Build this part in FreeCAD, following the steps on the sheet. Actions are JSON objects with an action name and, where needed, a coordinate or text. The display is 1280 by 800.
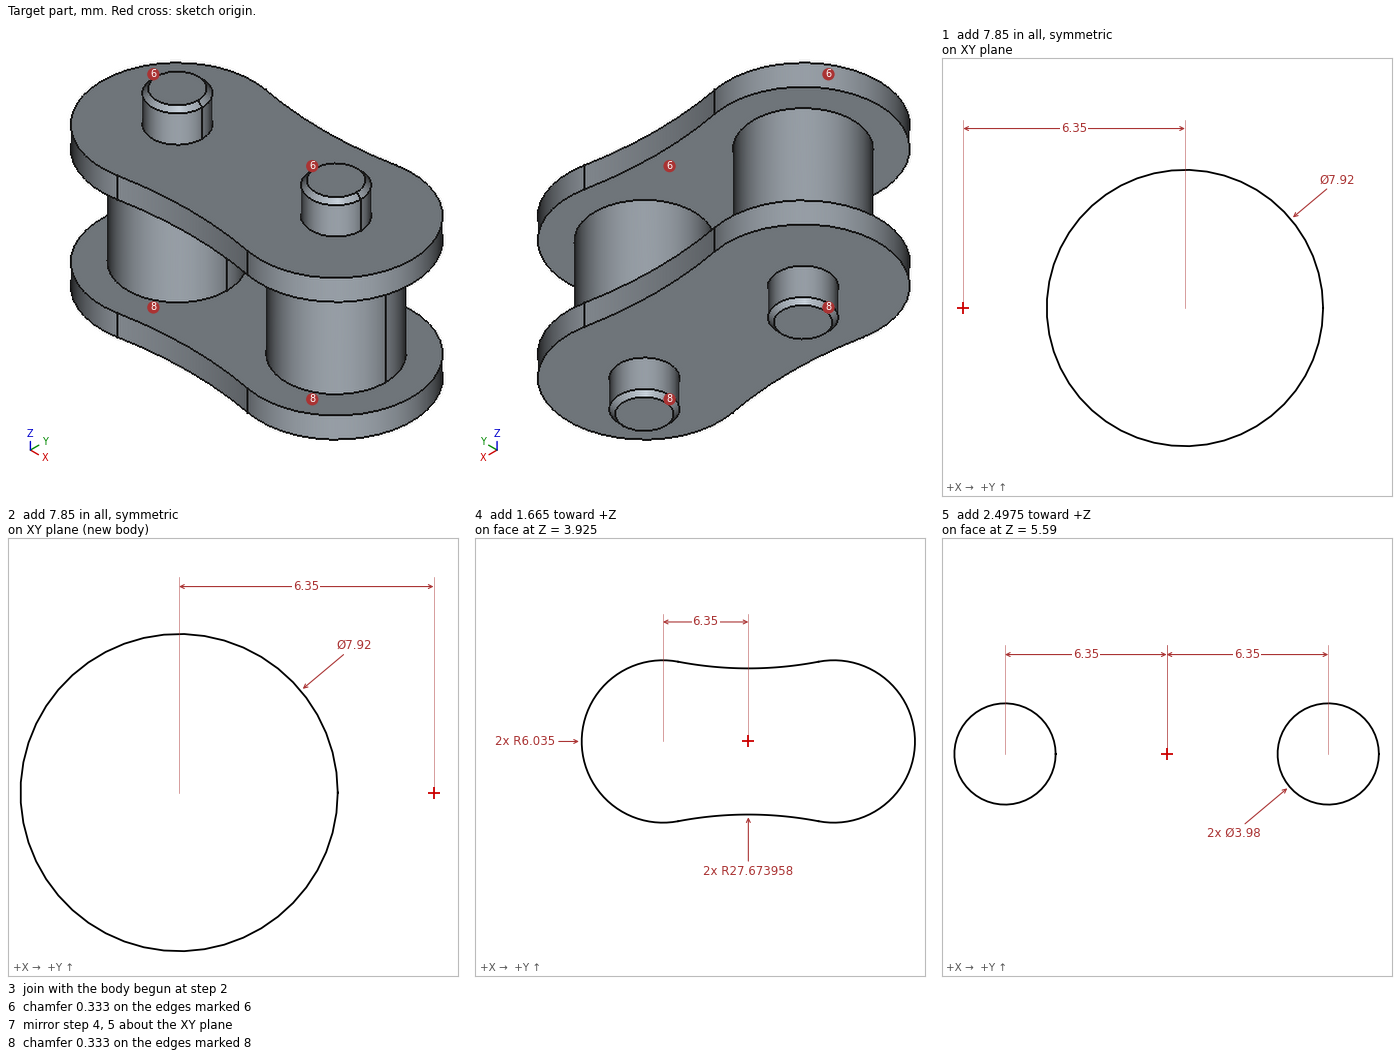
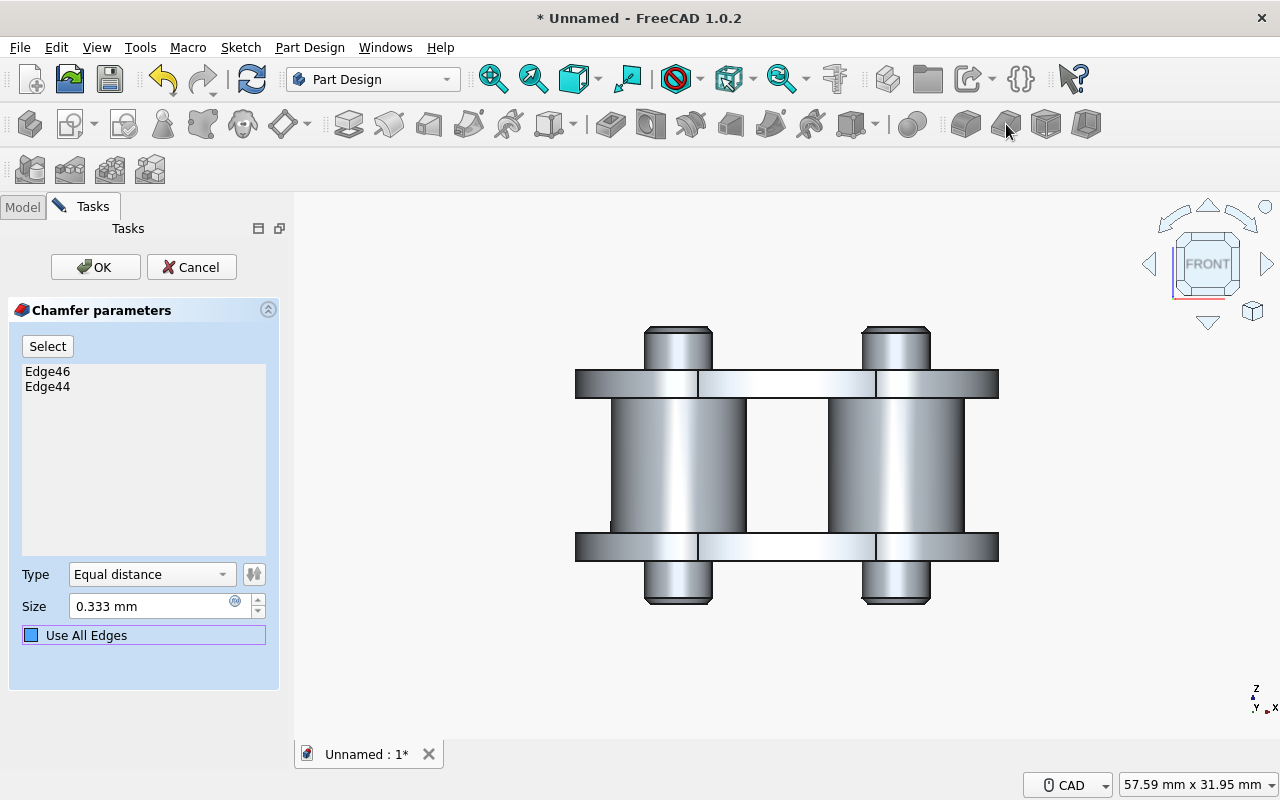
{"action": "left_click", "coordinate": [96, 267]}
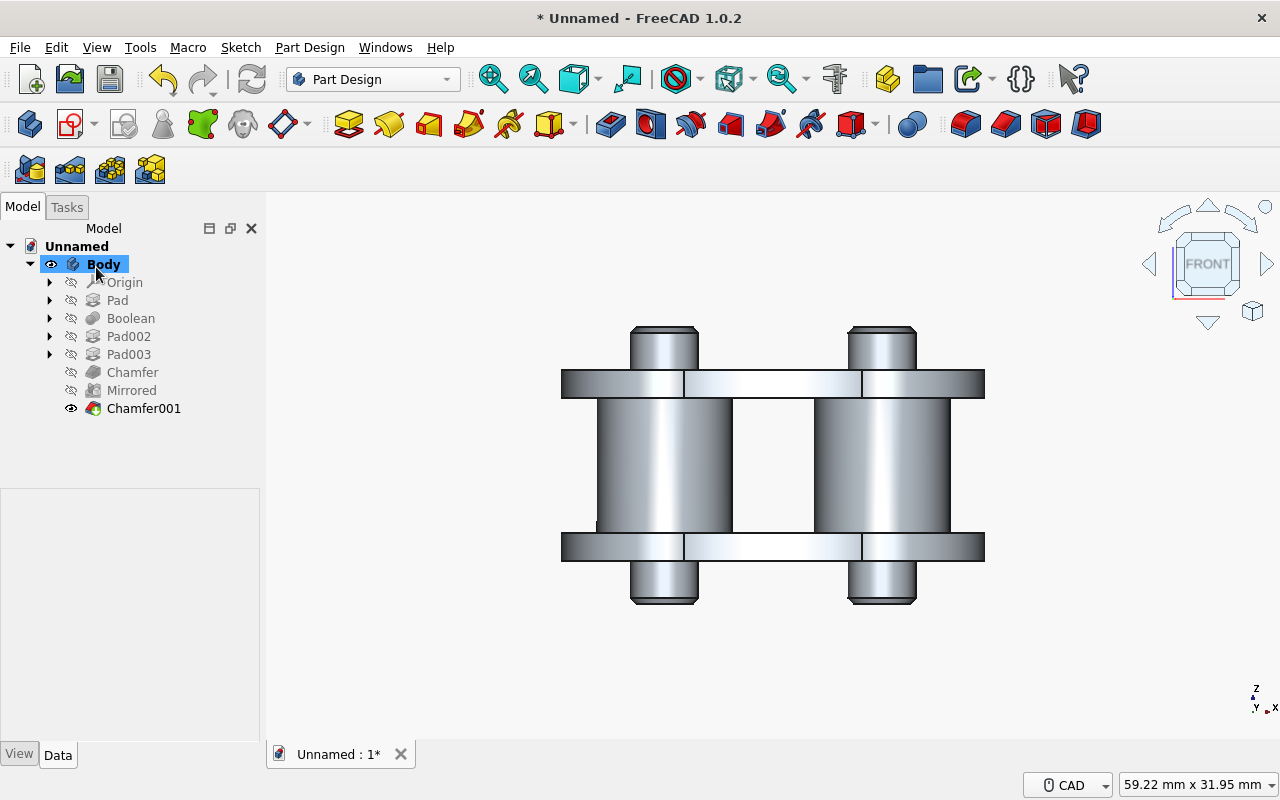
{"action": "key", "text": "0"}